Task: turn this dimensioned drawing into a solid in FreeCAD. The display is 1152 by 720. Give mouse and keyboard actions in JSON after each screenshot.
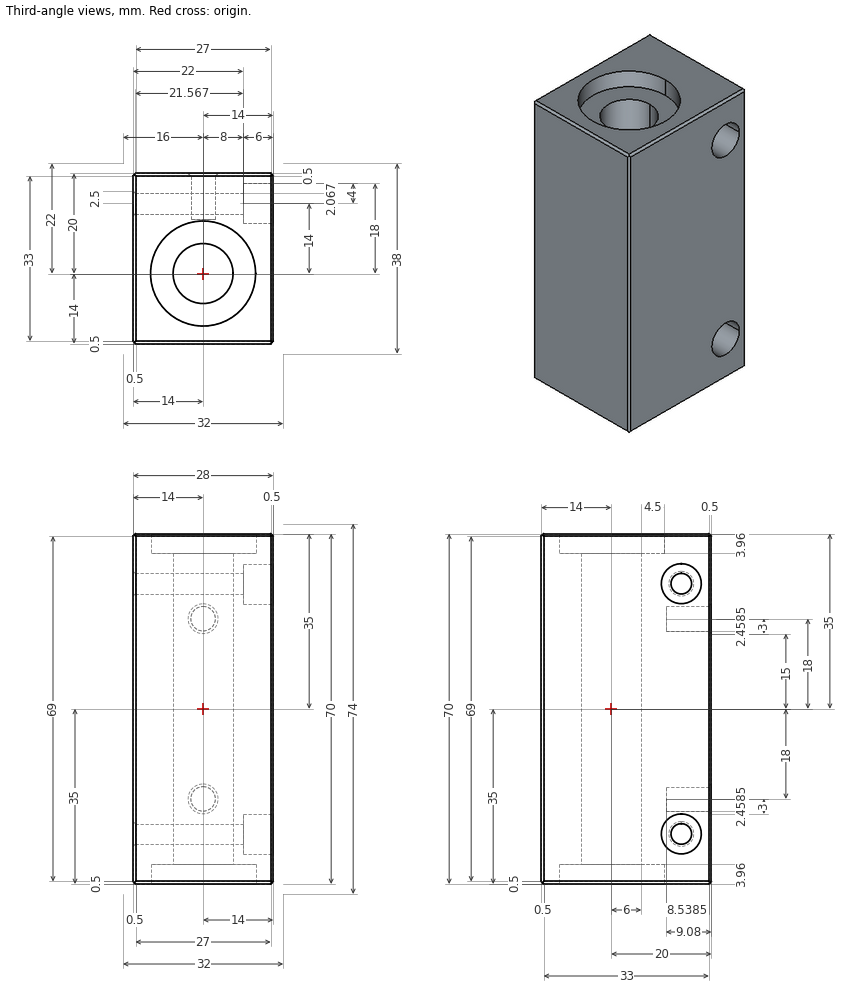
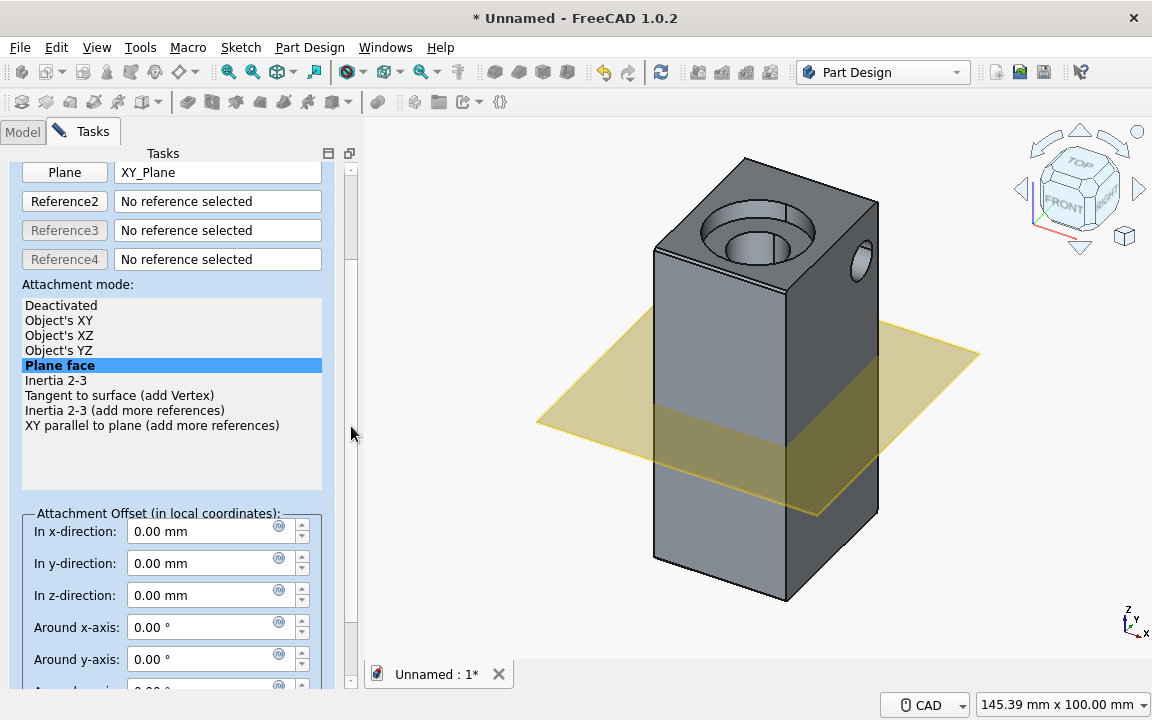
{"action": "triple_click", "coordinate": [210, 595]}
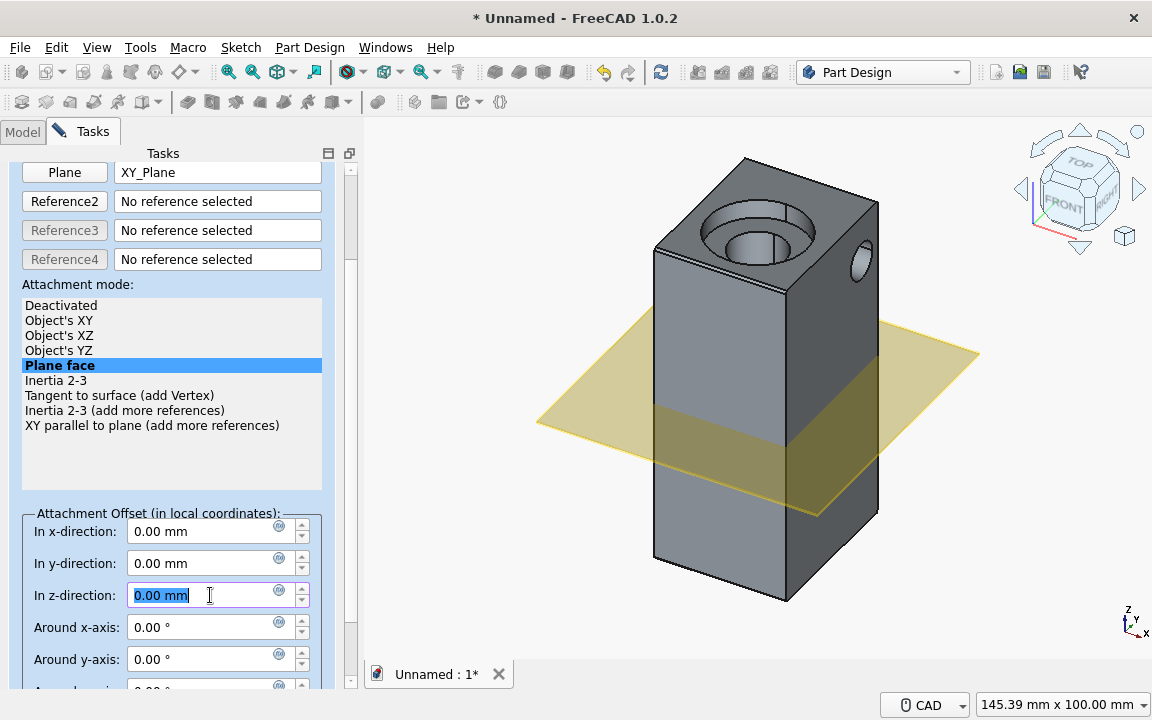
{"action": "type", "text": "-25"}
{"action": "key", "text": "Tab"}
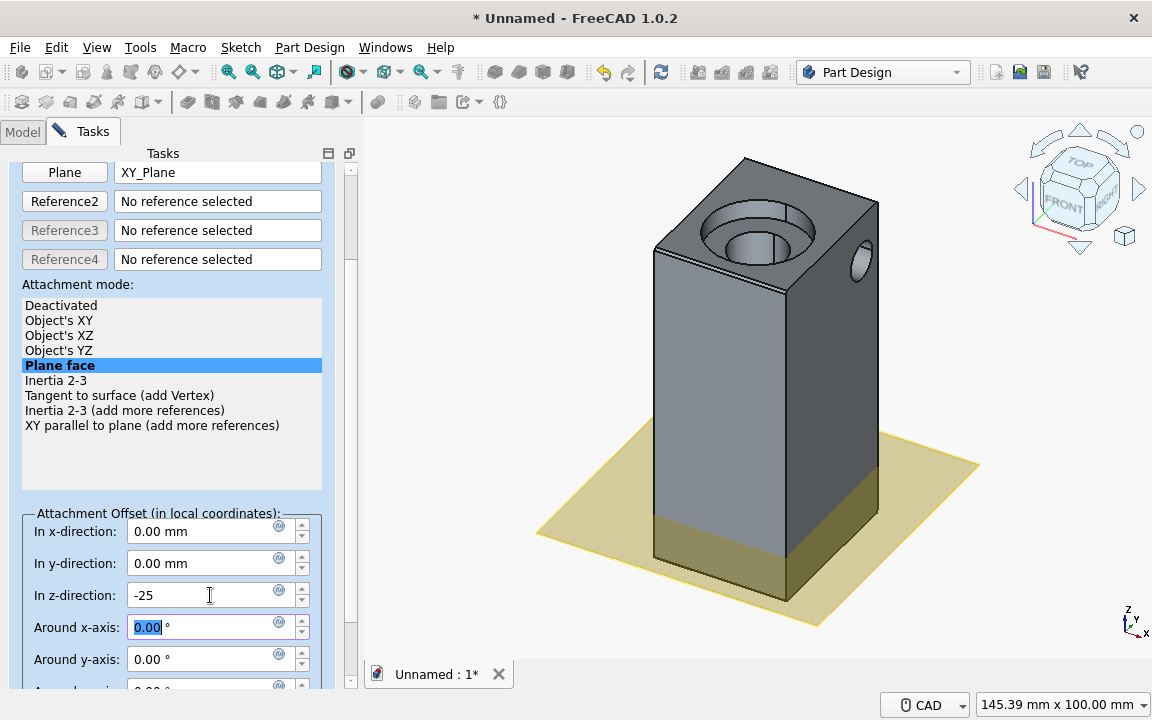
{"action": "scroll", "coordinate": [351, 426], "scroll_direction": "up", "scroll_amount": 3}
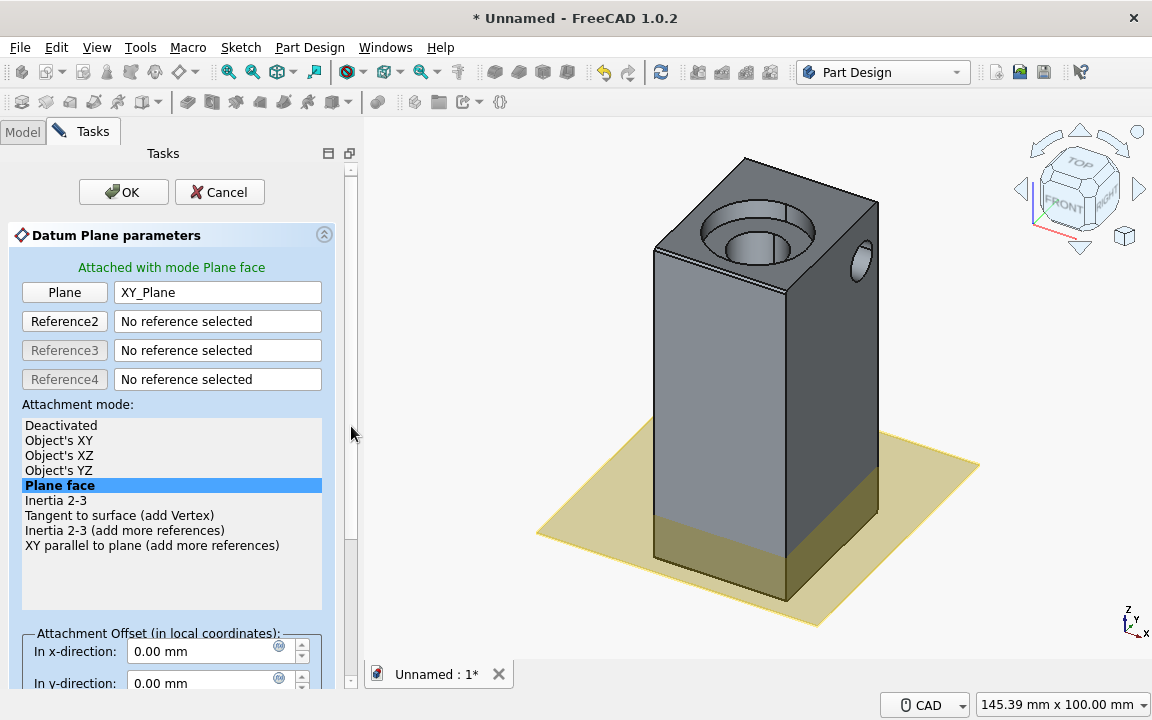
{"action": "left_click", "coordinate": [124, 192]}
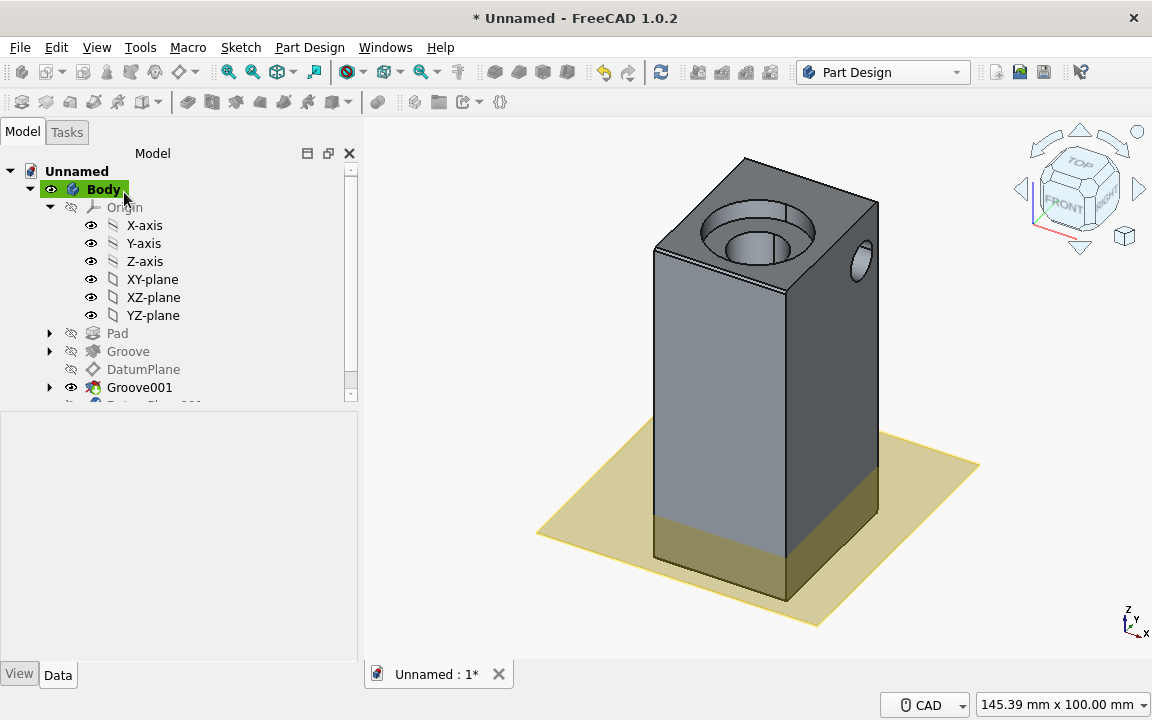
{"action": "scroll", "coordinate": [100, 275], "scroll_direction": "down", "scroll_amount": 3}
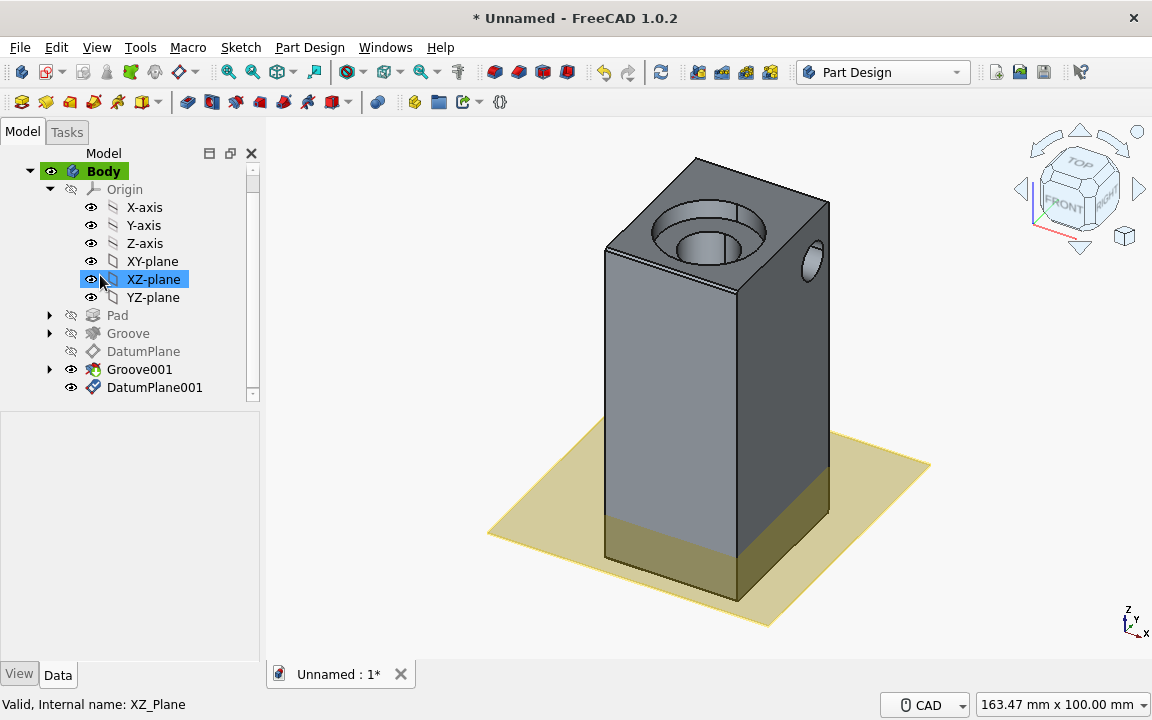
{"action": "left_click", "coordinate": [116, 387]}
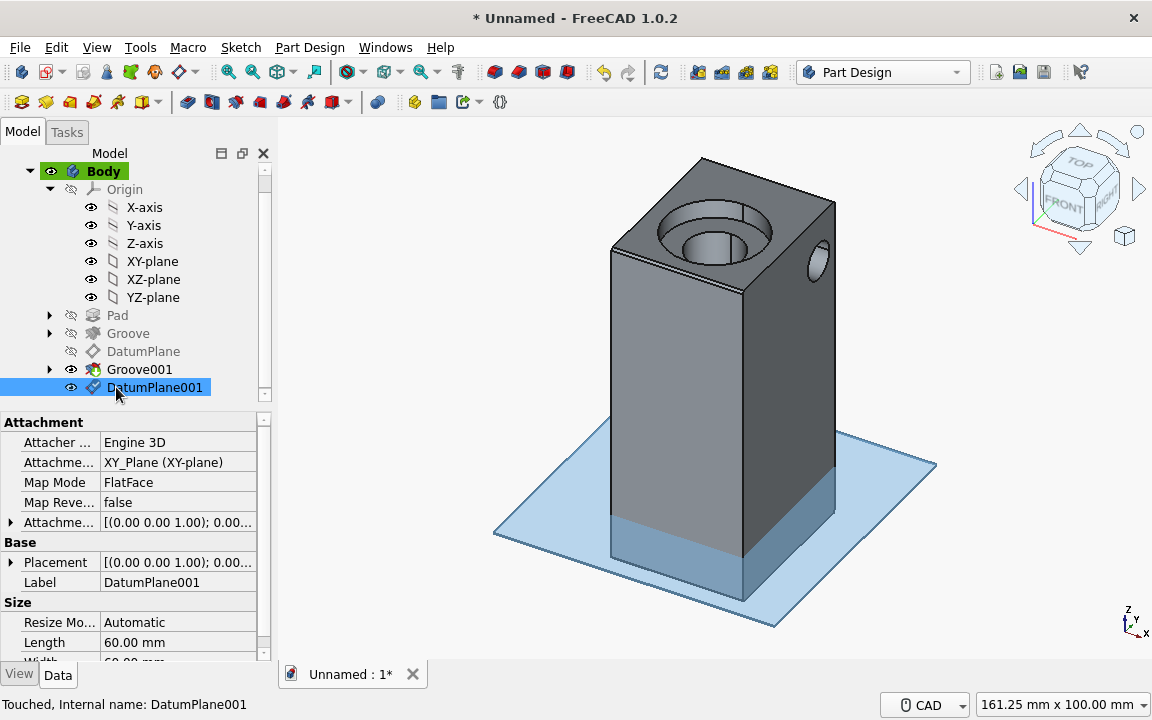
{"action": "left_click", "coordinate": [46, 72]}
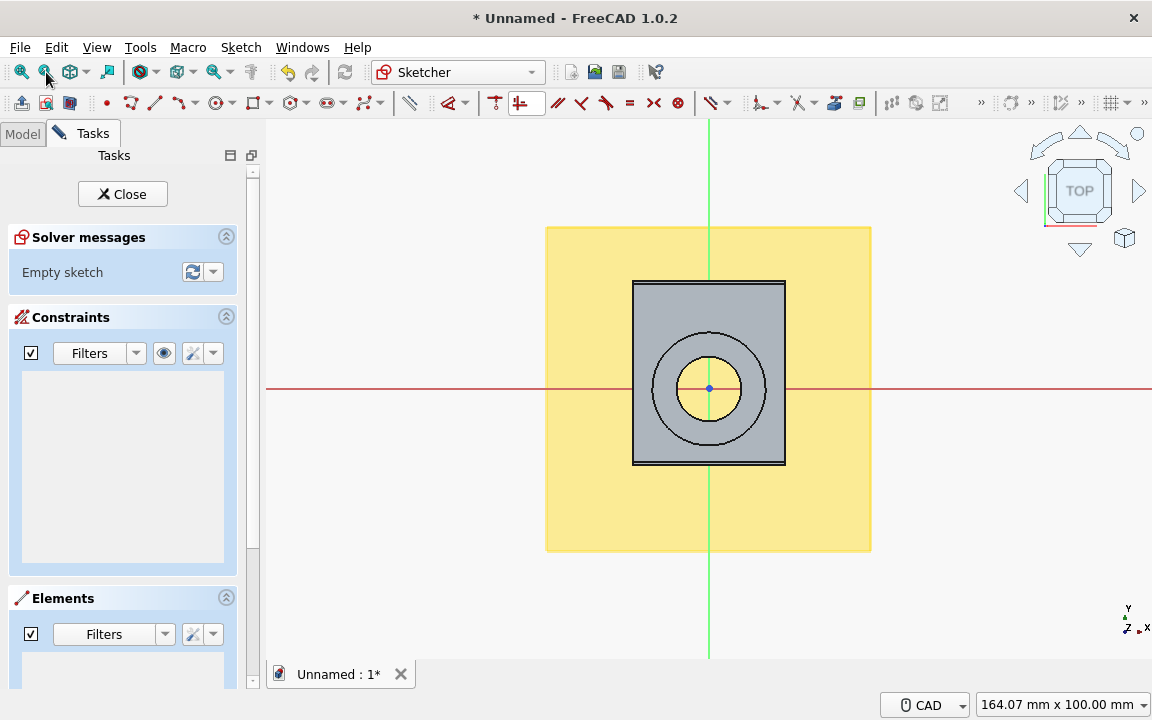
{"action": "left_click", "coordinate": [70, 104]}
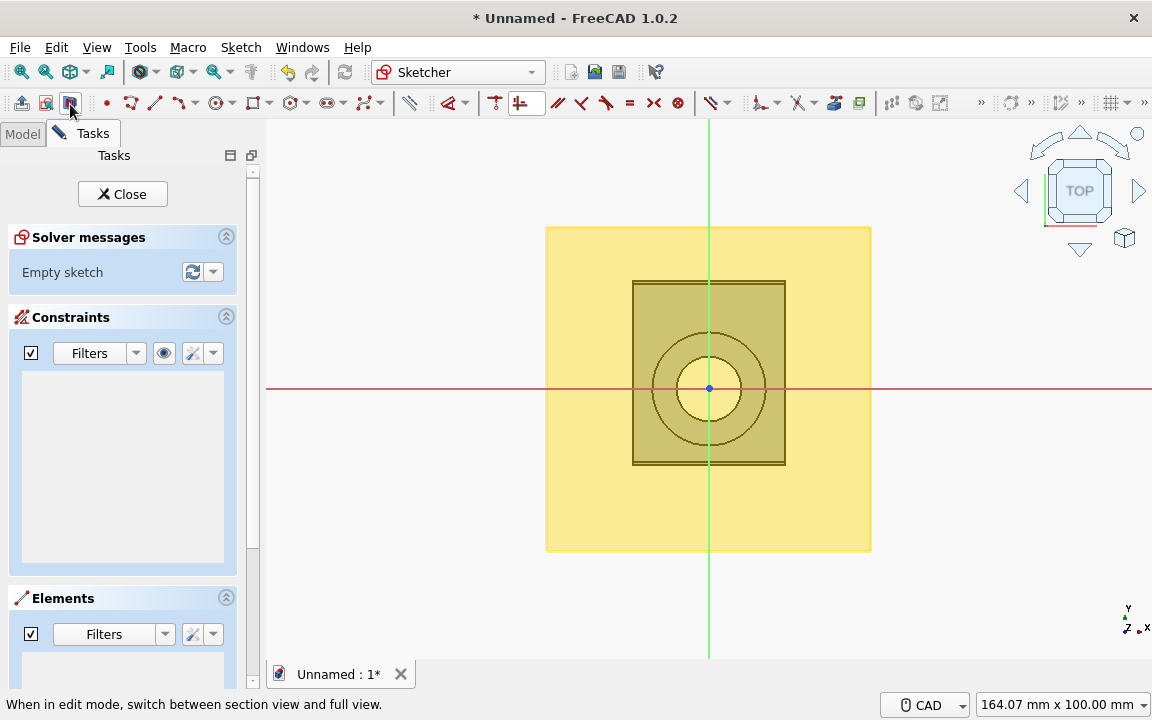
{"action": "scroll", "coordinate": [793, 319], "scroll_direction": "up", "scroll_amount": 6}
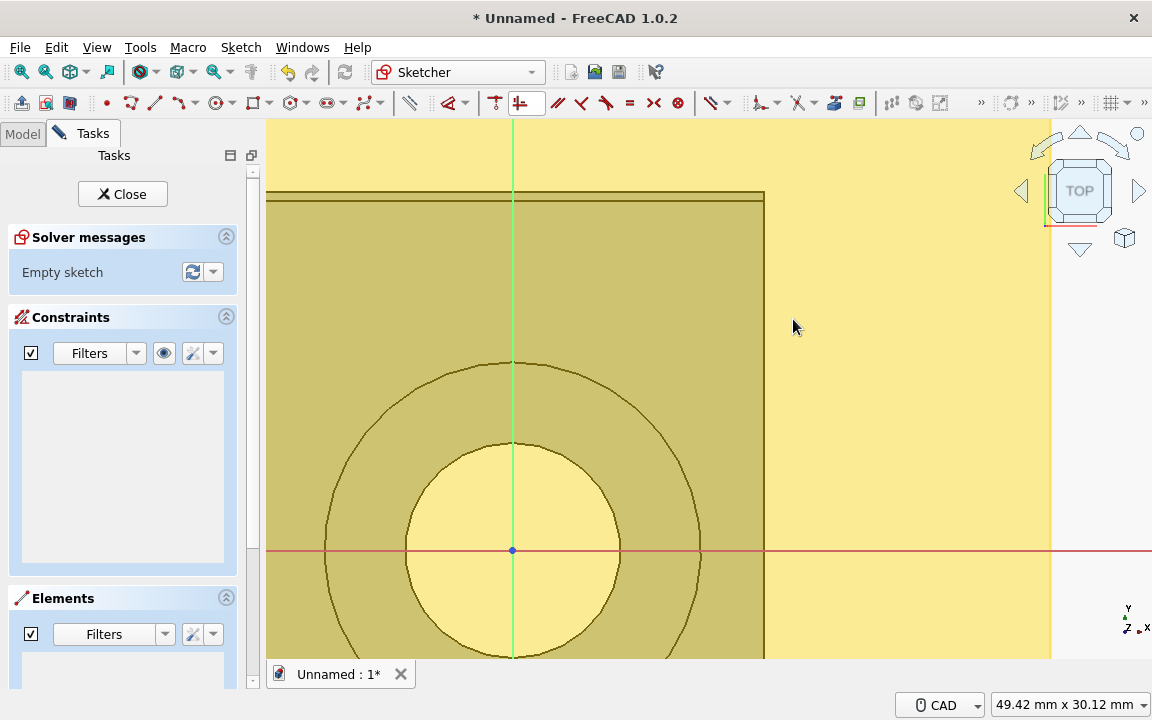
{"action": "left_click", "coordinate": [254, 104]}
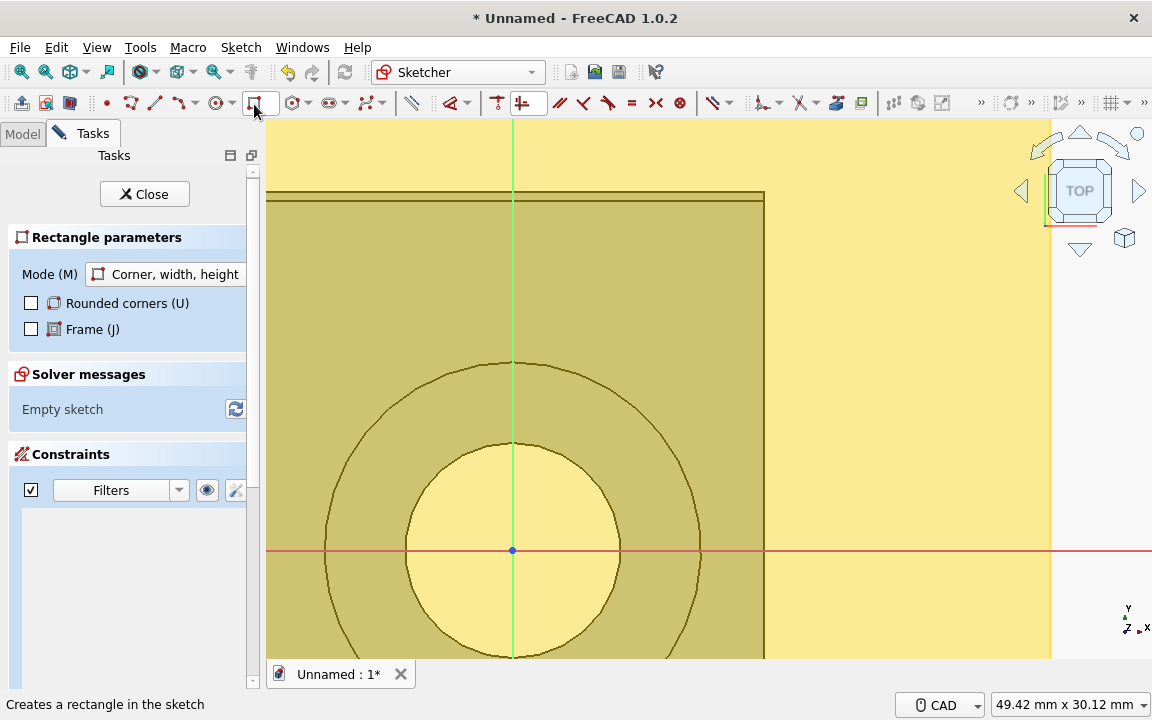
{"action": "left_click", "coordinate": [656, 228]}
{"action": "mouse_move", "coordinate": [764, 300]}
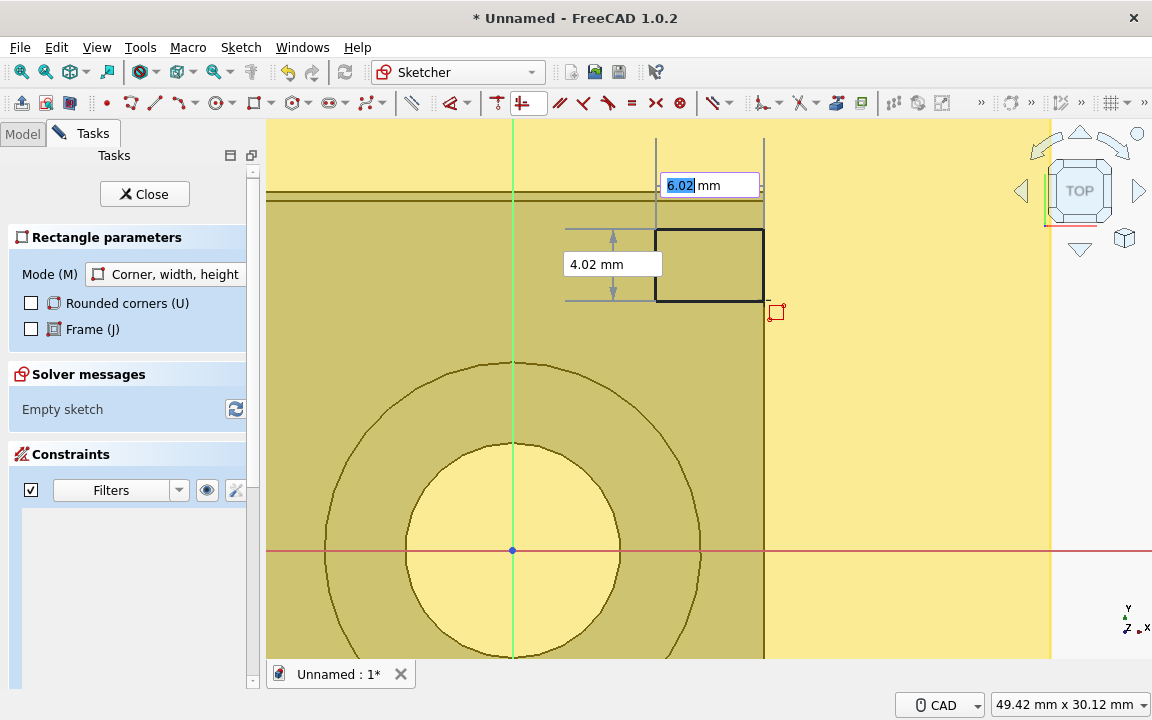
{"action": "type", "text": "6"}
{"action": "key", "text": "Tab"}
{"action": "type", "text": "4"}
{"action": "key", "text": "Return"}